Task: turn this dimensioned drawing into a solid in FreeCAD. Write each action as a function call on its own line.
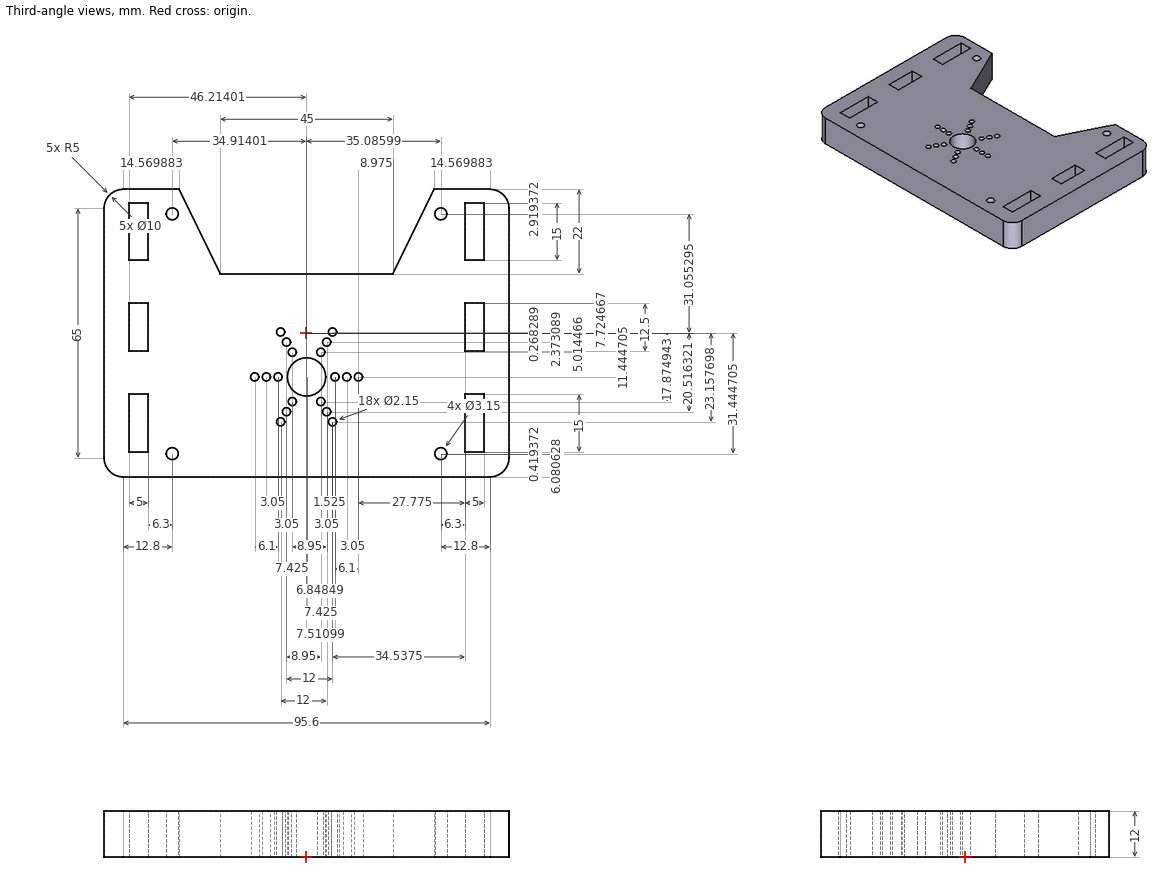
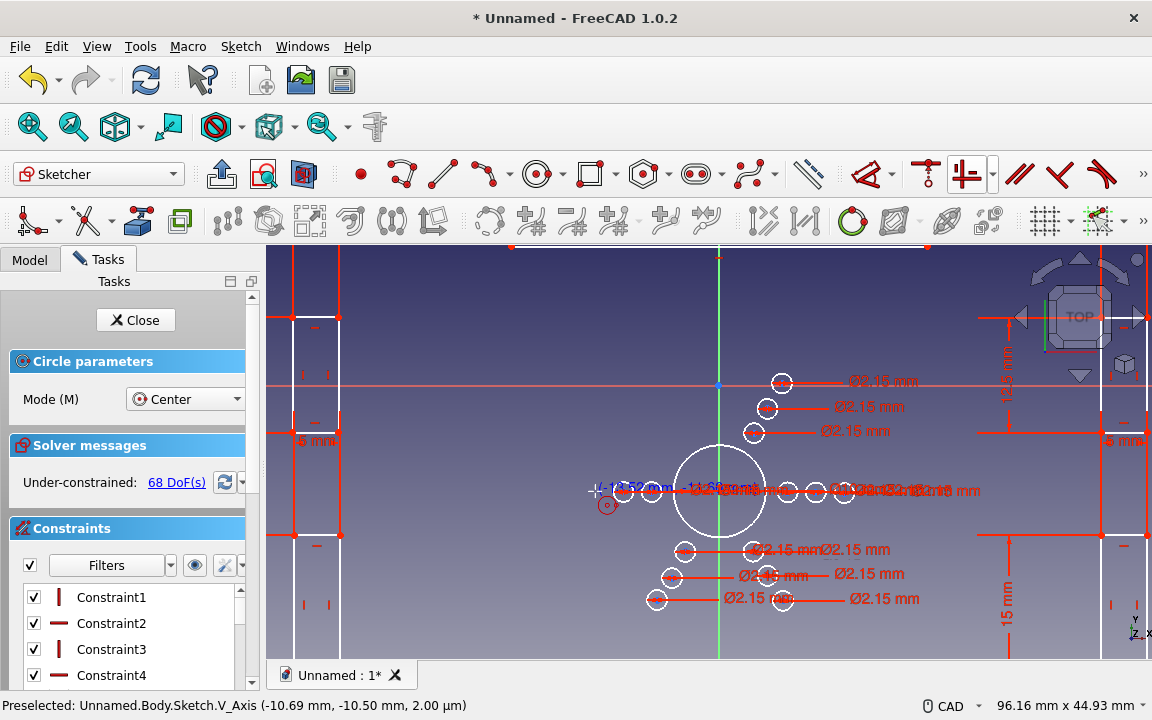
click(595, 491)
move(588, 484)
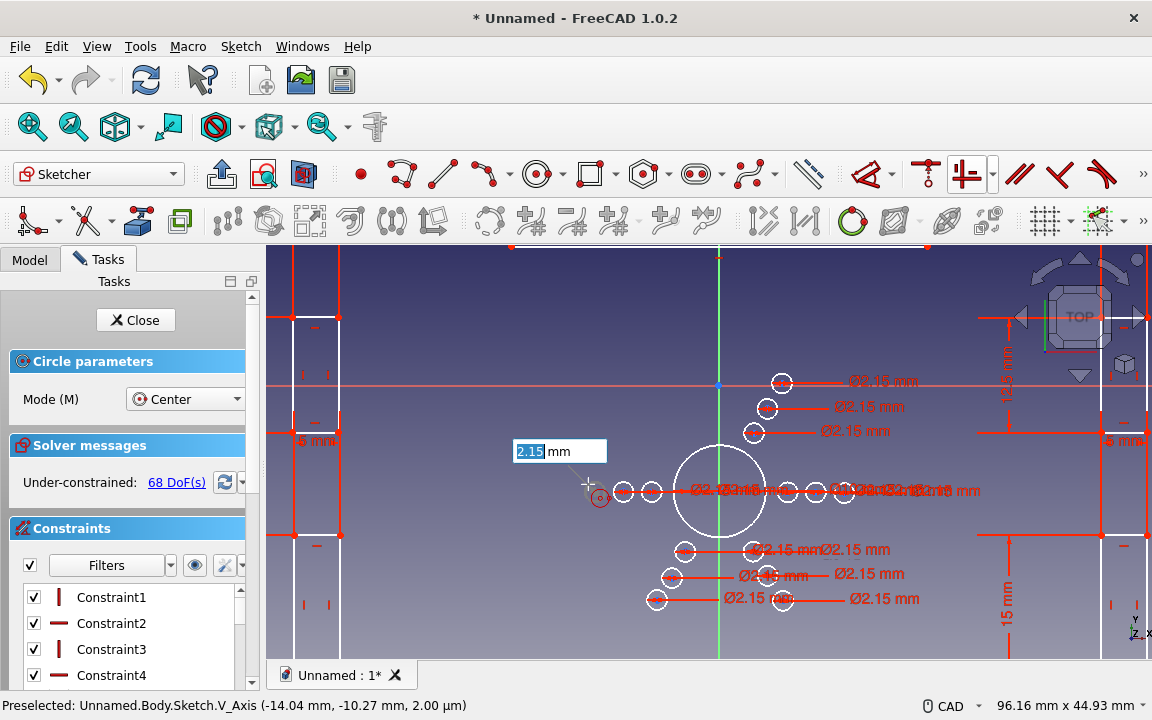
text(2.15)
key(Return)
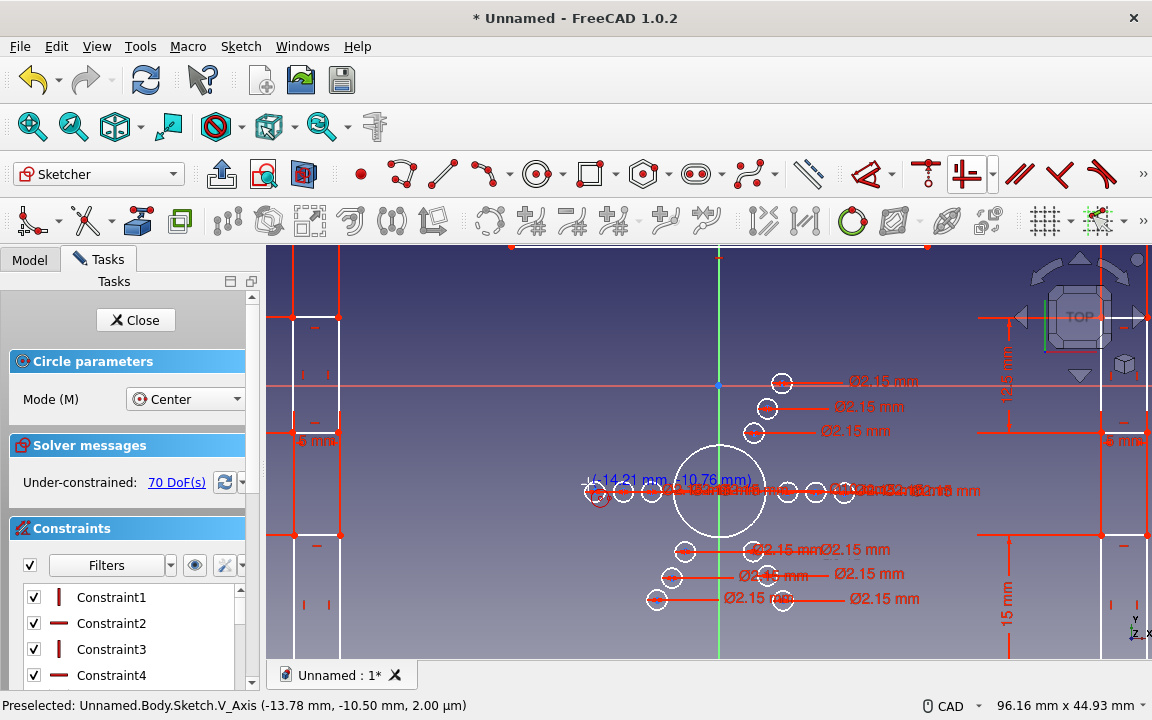
scroll(685, 432, up, 5)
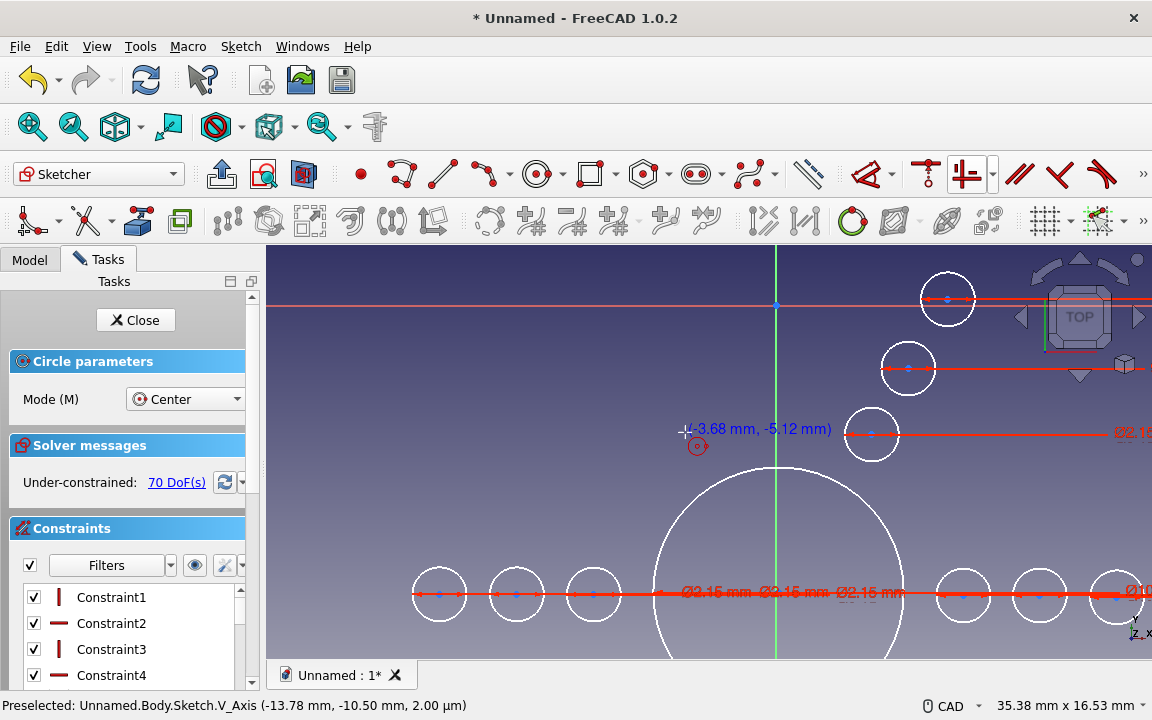
scroll(619, 475, down, 10)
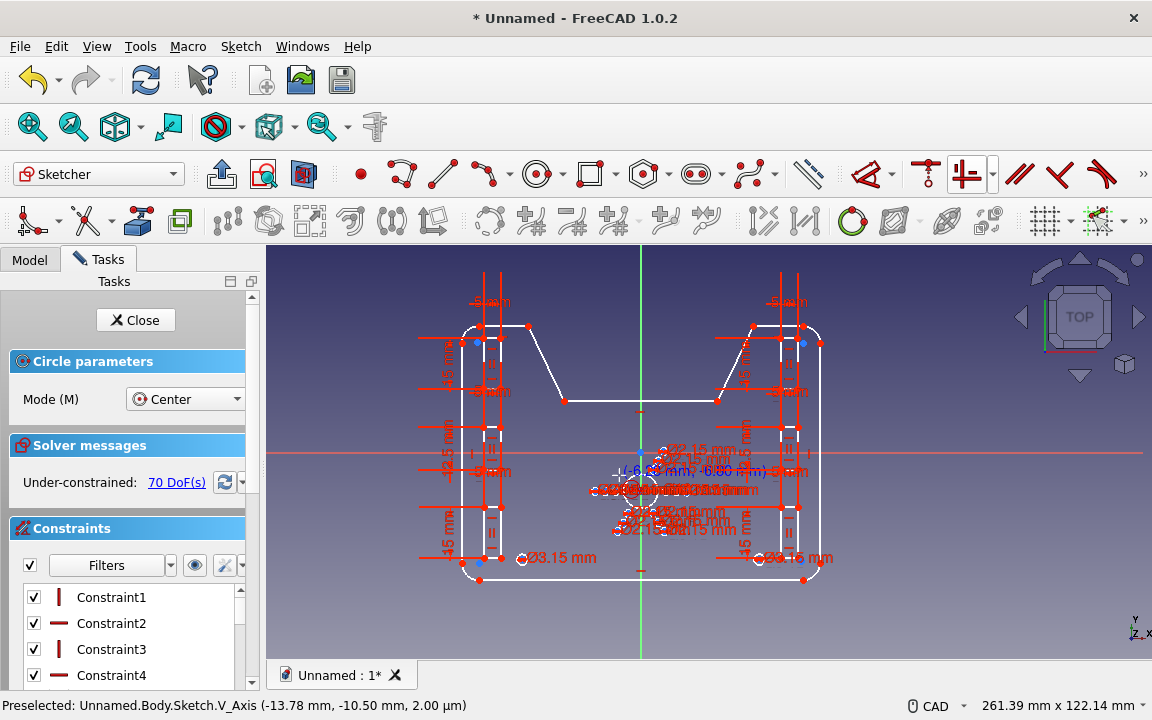
scroll(628, 470, up, 4)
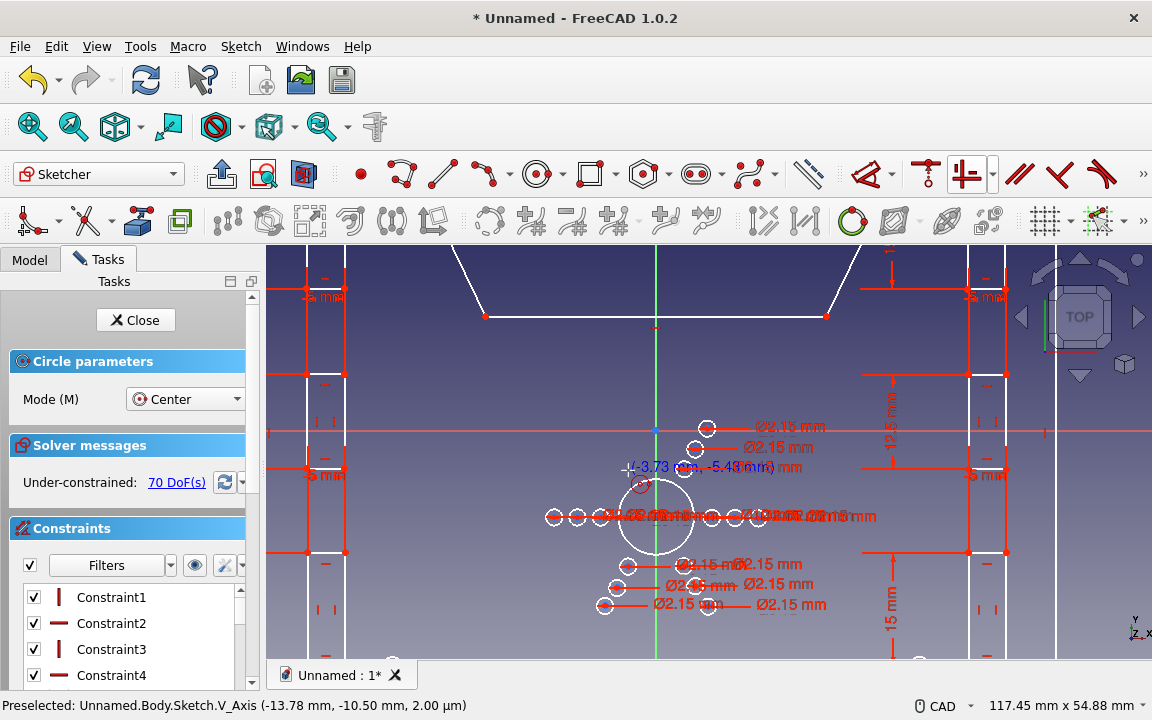
click(628, 468)
move(634, 463)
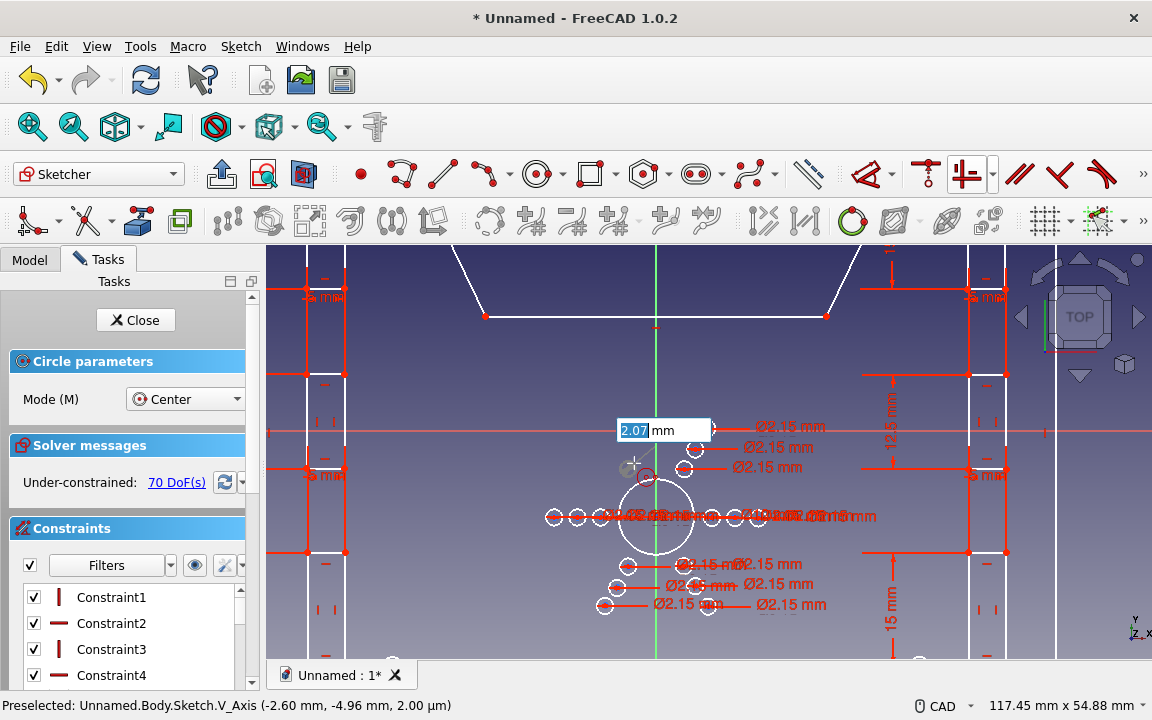
text(2.15)
key(Return)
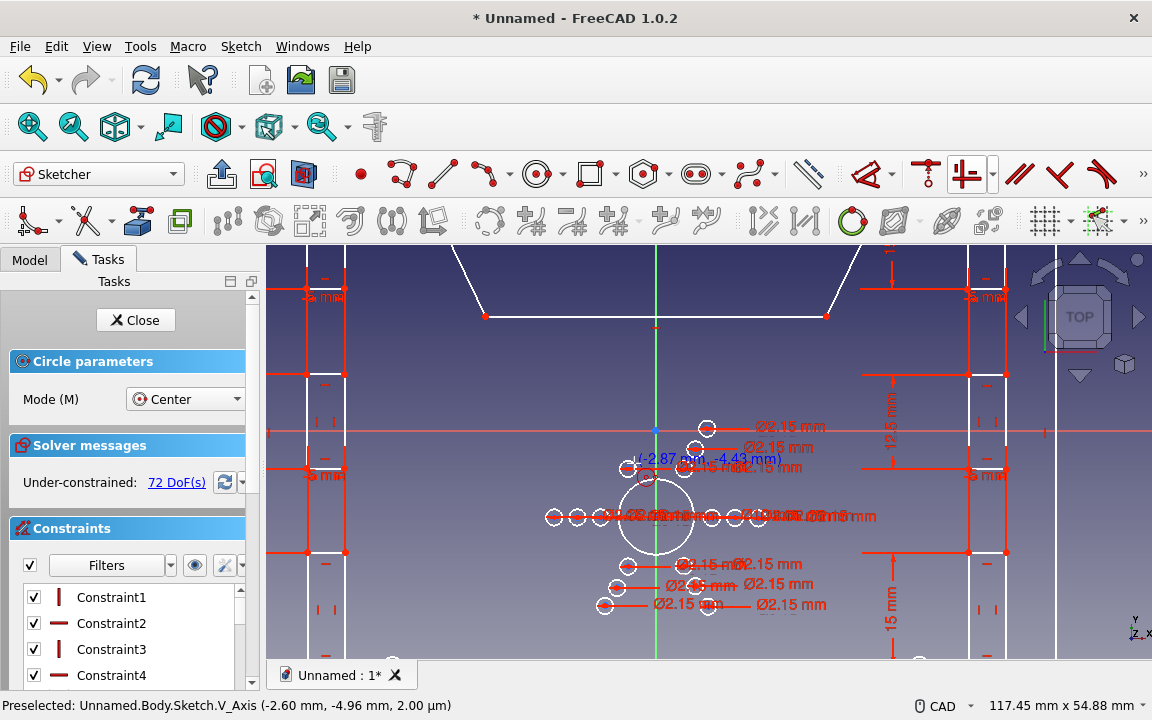
scroll(617, 448, up, 6)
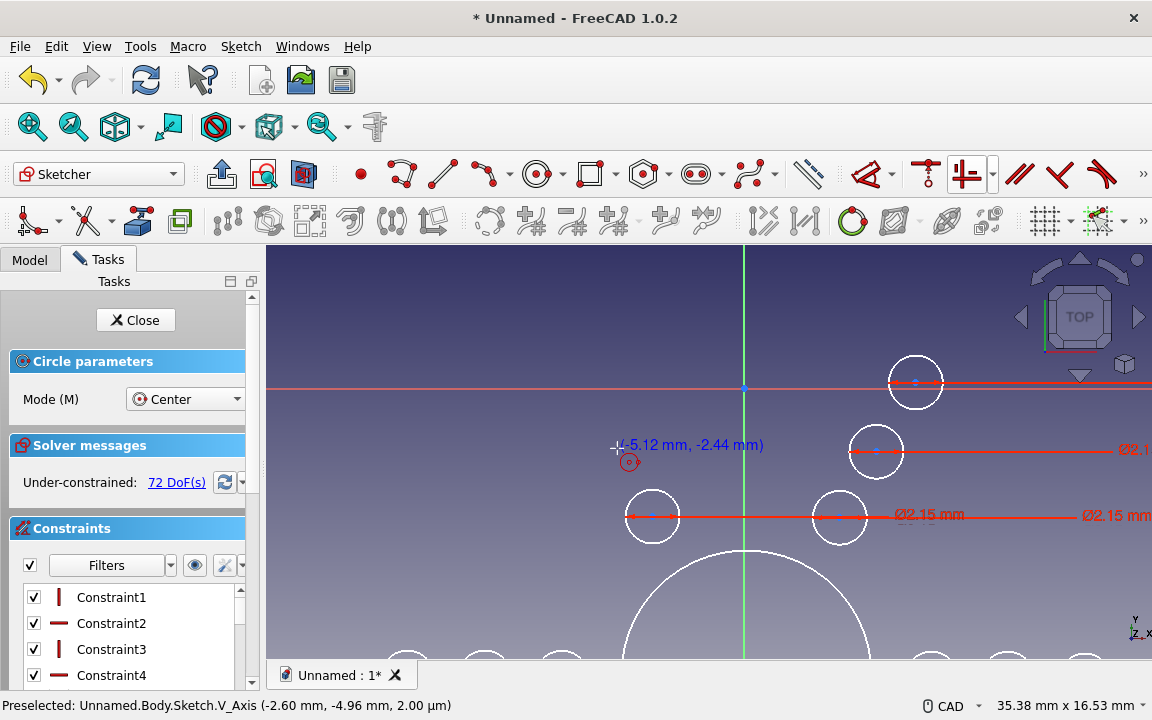
scroll(624, 462, down, 10)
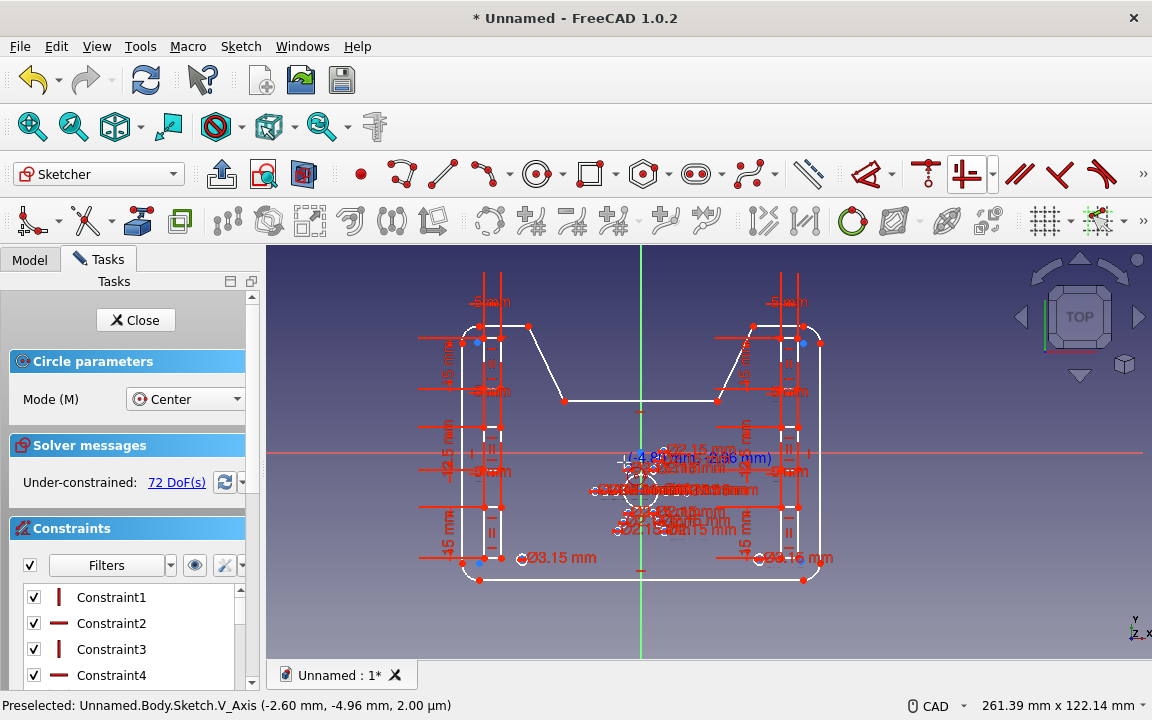
scroll(623, 461, up, 5)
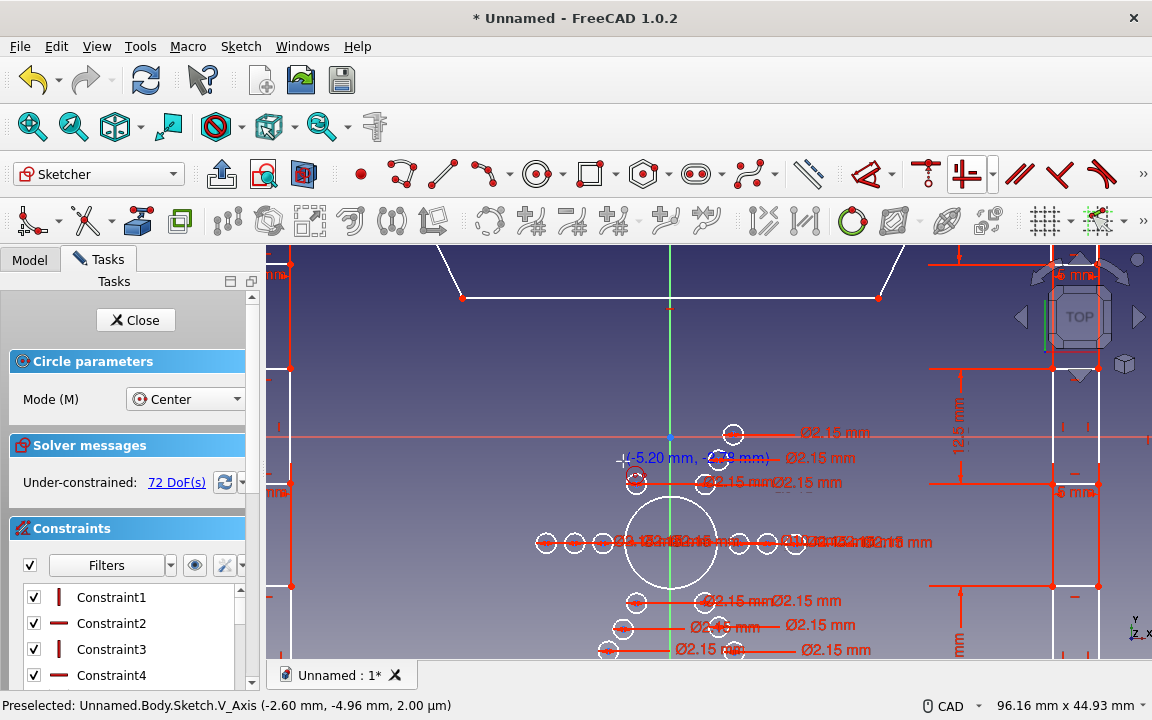
click(623, 459)
move(630, 452)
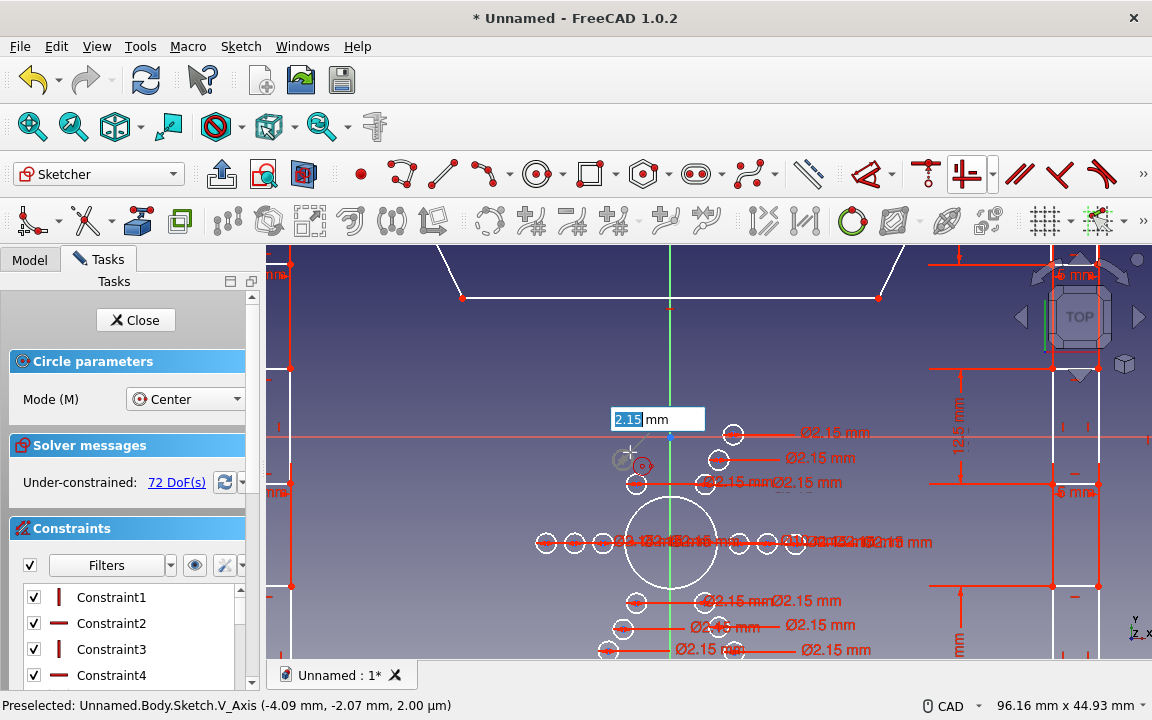
text(2.15)
key(Return)